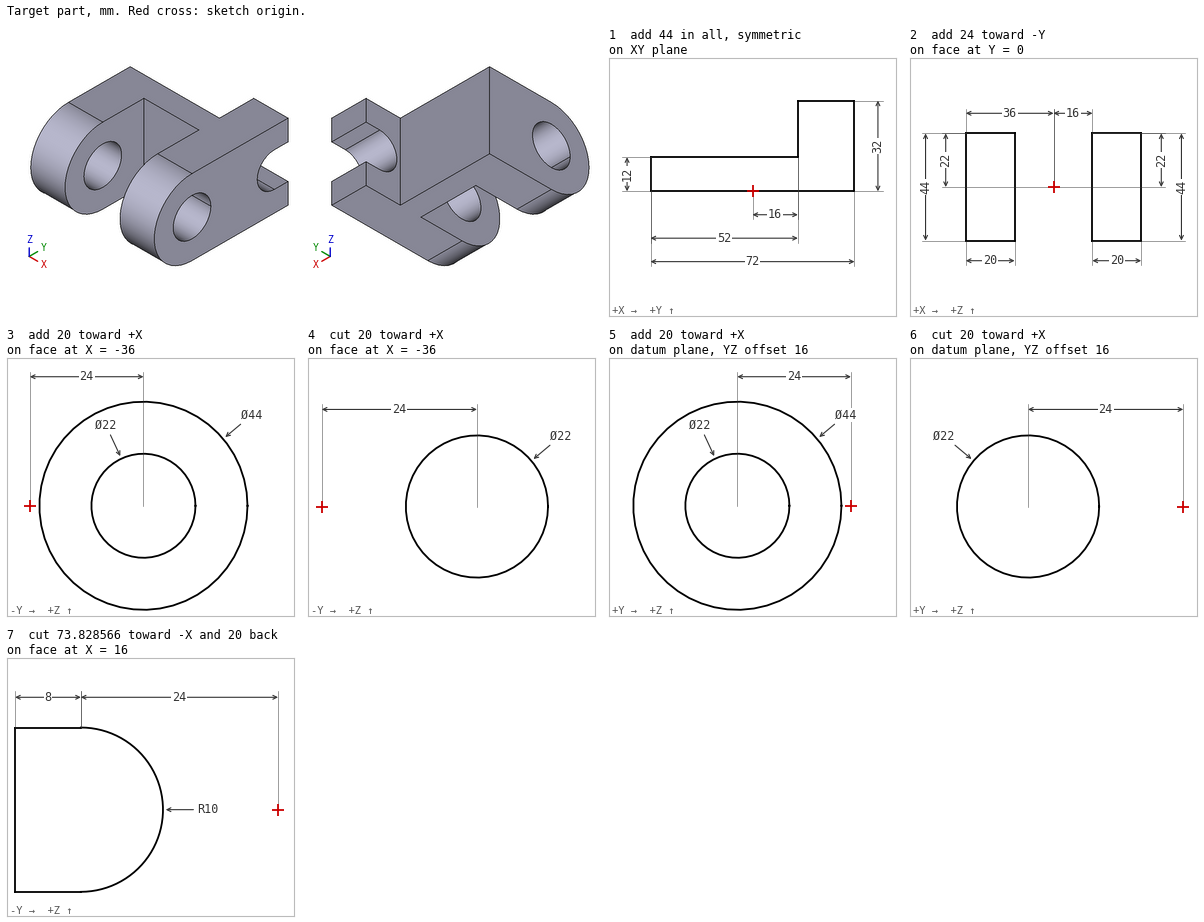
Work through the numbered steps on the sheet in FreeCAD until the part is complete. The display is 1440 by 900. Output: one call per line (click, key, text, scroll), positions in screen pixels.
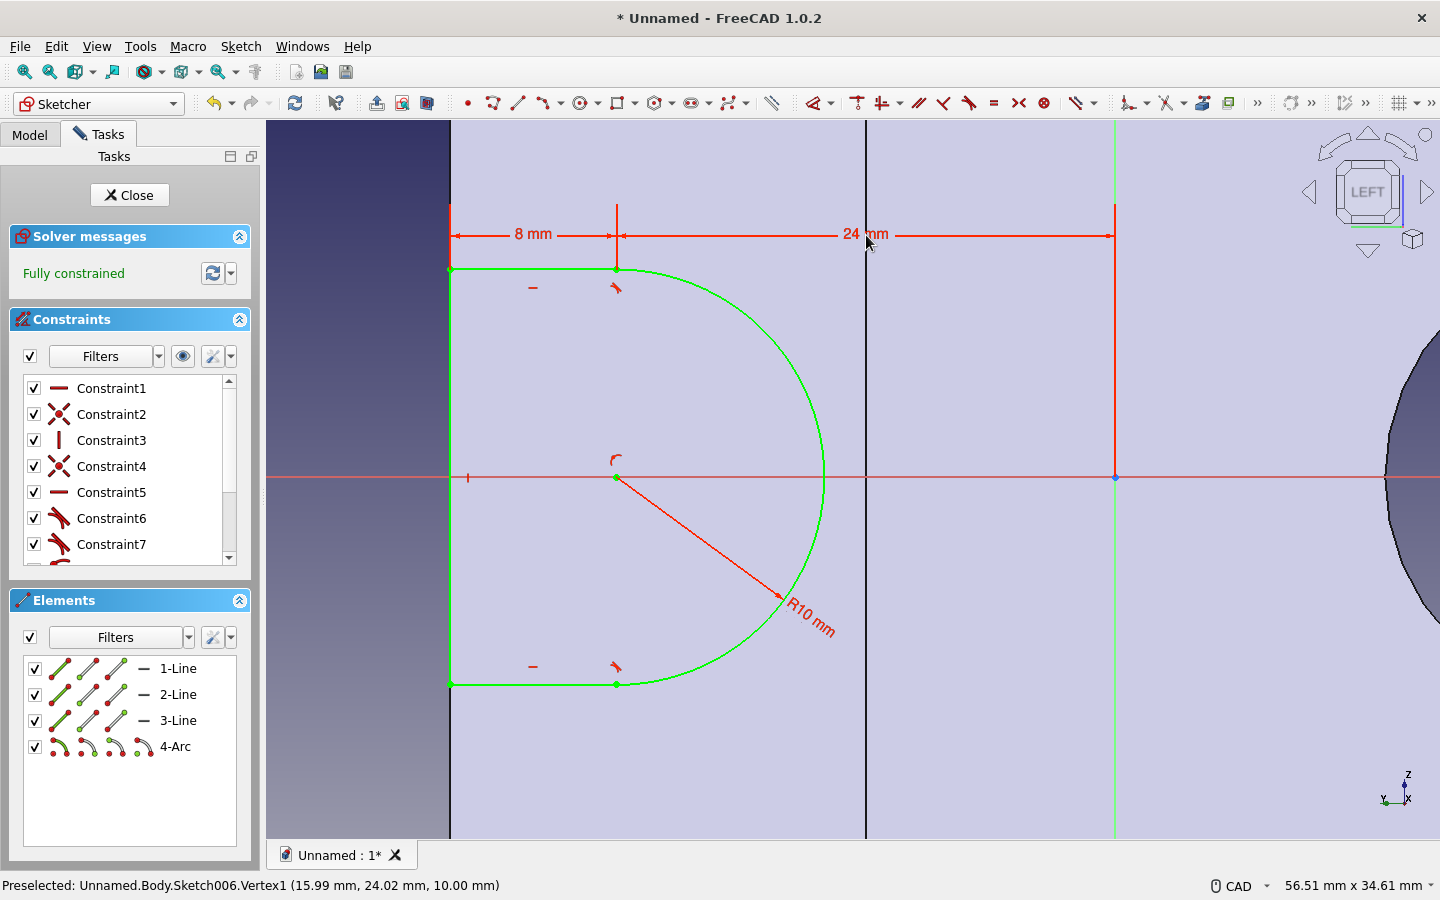
click(130, 195)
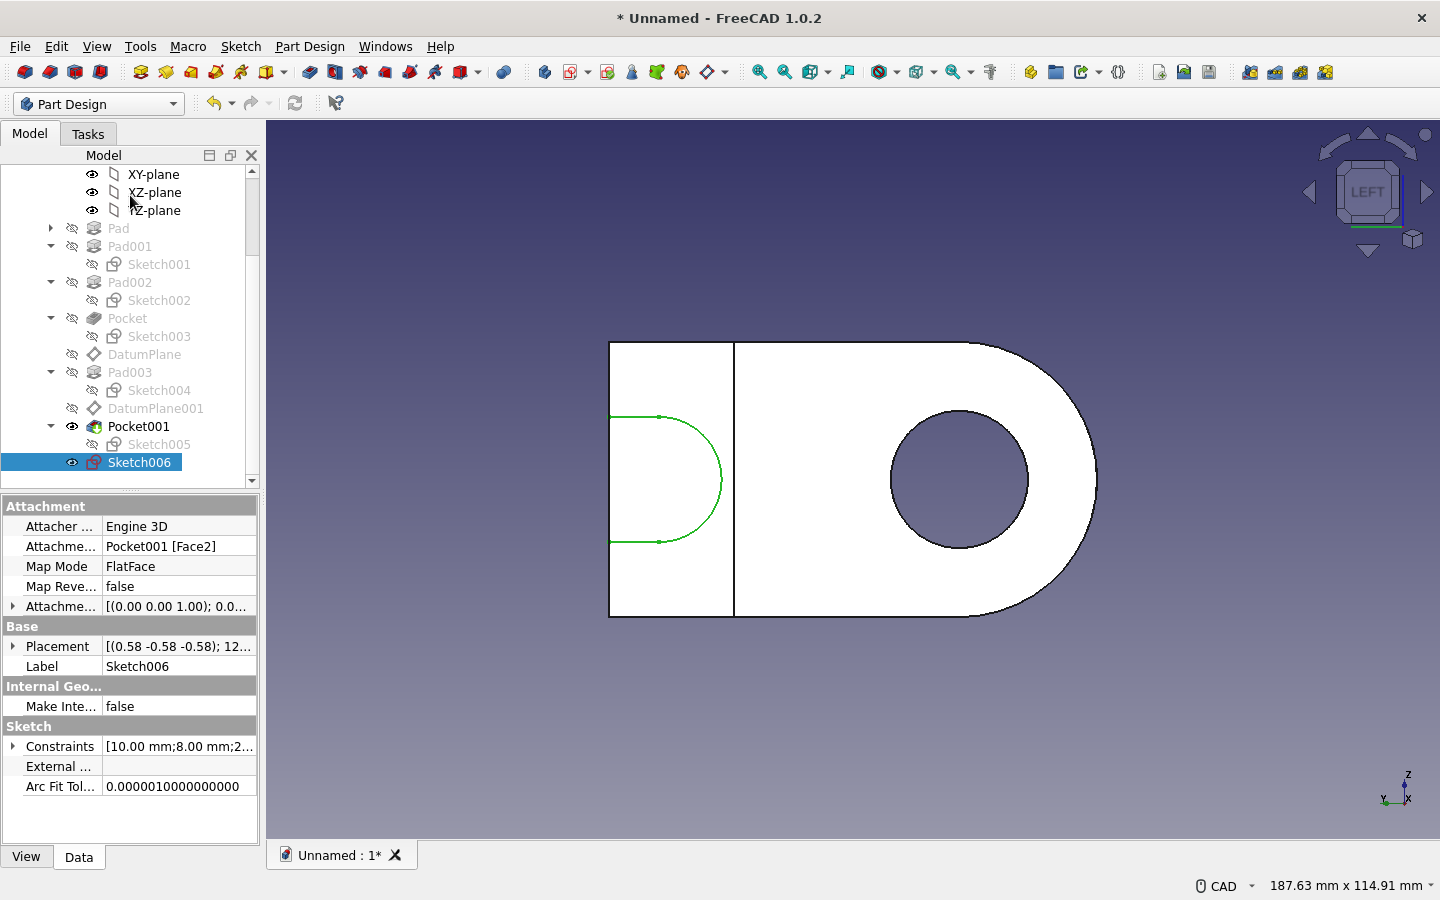
click(310, 72)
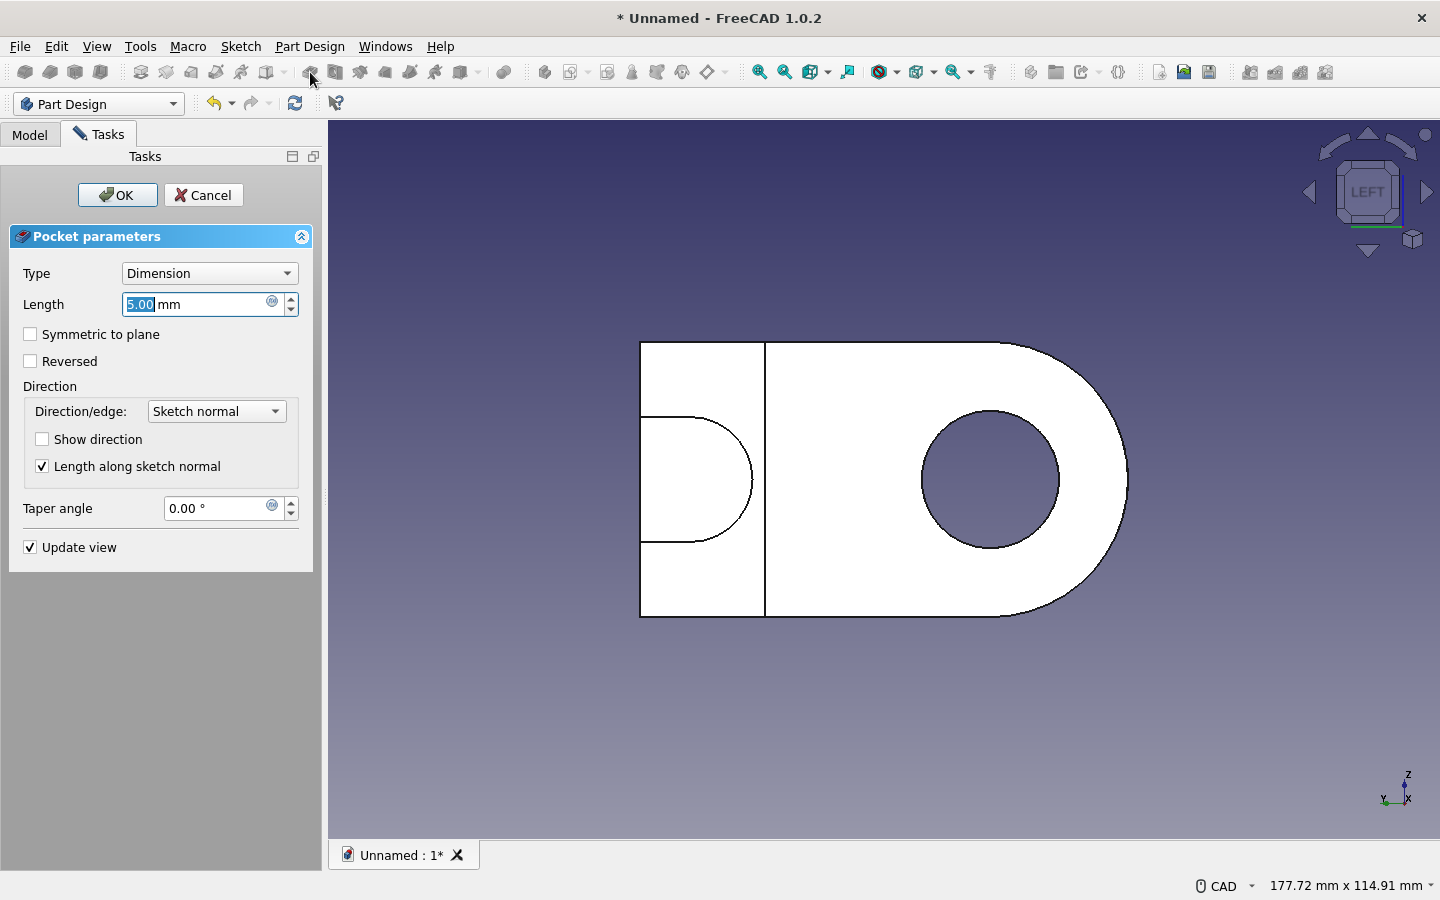
click(210, 274)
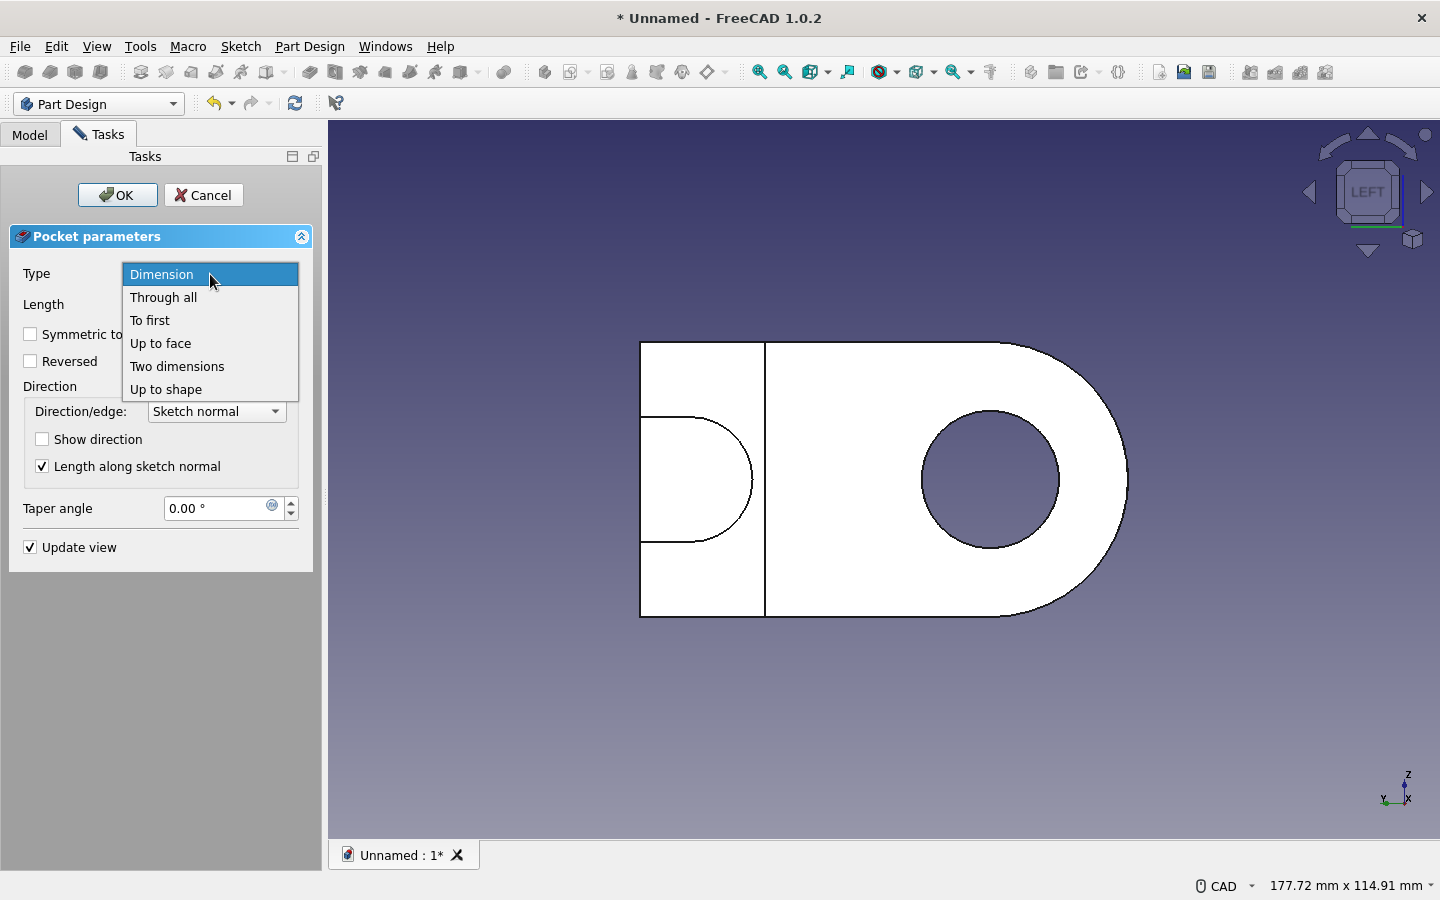
click(208, 366)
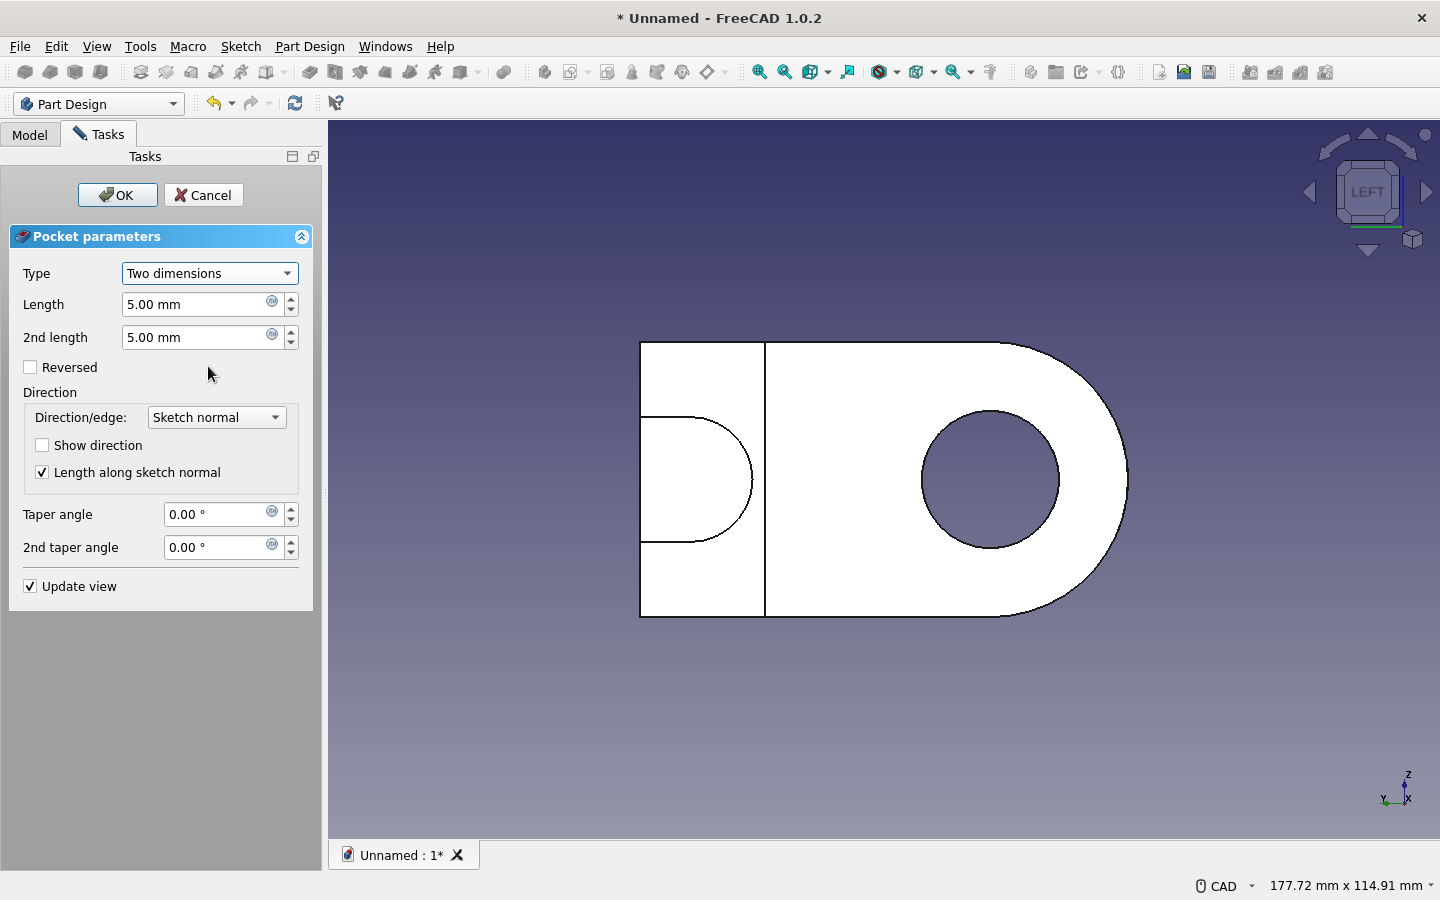
triple_click(204, 304)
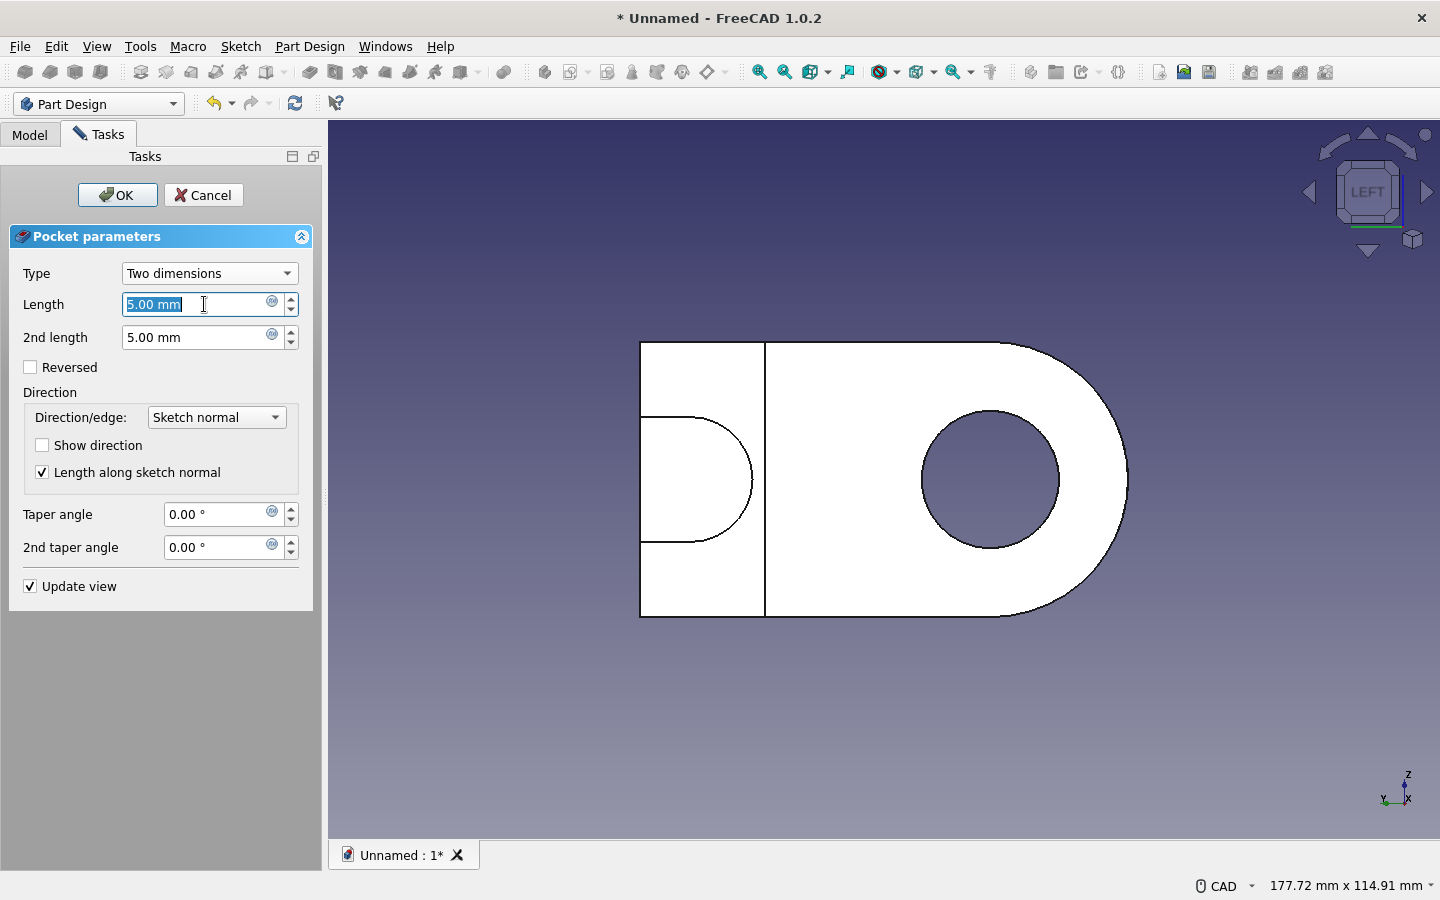
text(73.828566)
key(Tab)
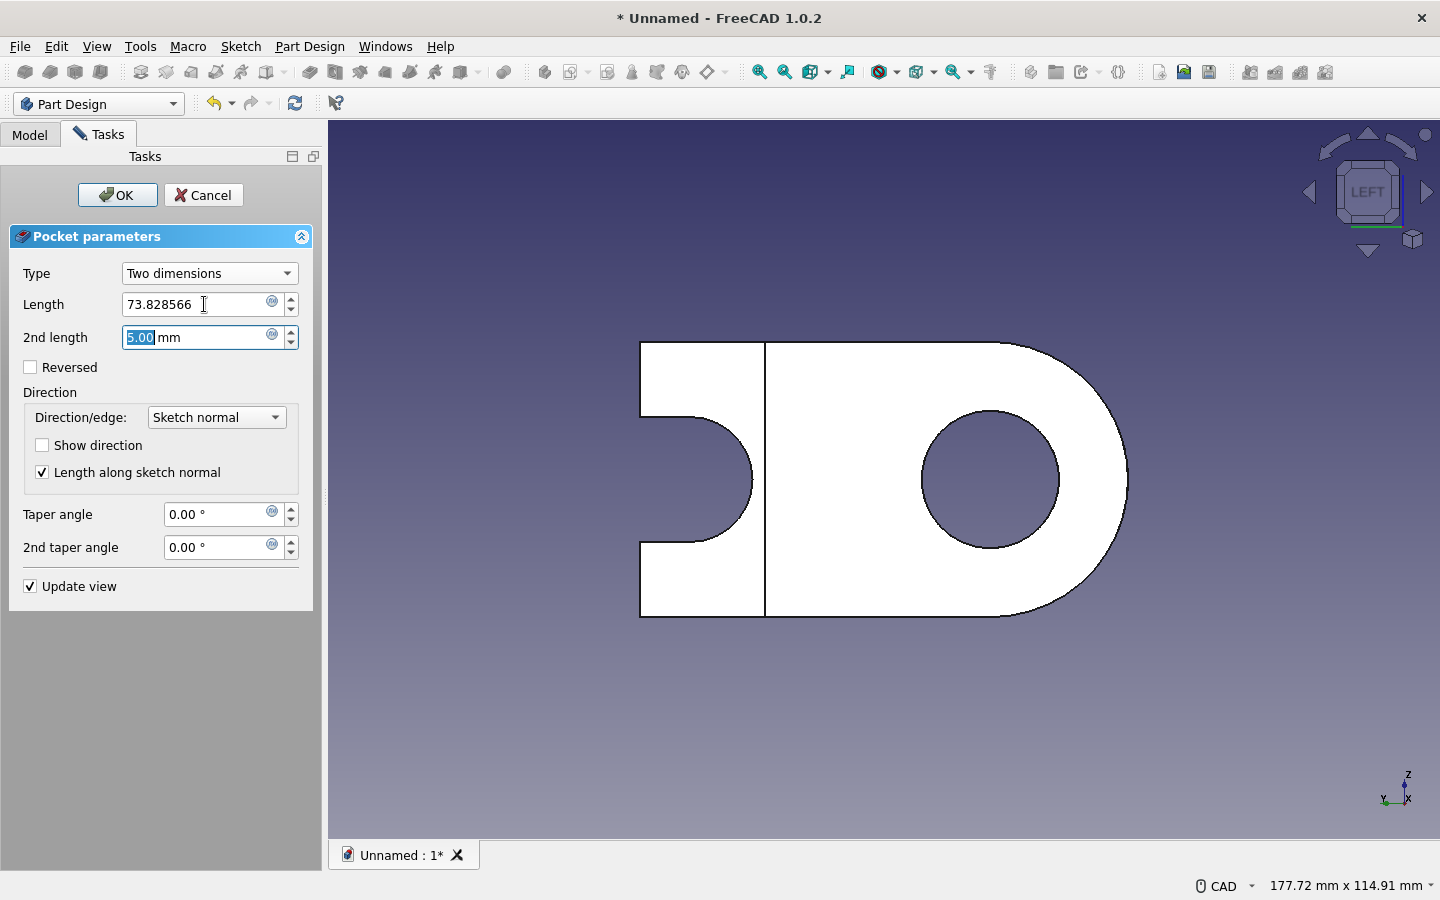
text(20)
key(Tab)